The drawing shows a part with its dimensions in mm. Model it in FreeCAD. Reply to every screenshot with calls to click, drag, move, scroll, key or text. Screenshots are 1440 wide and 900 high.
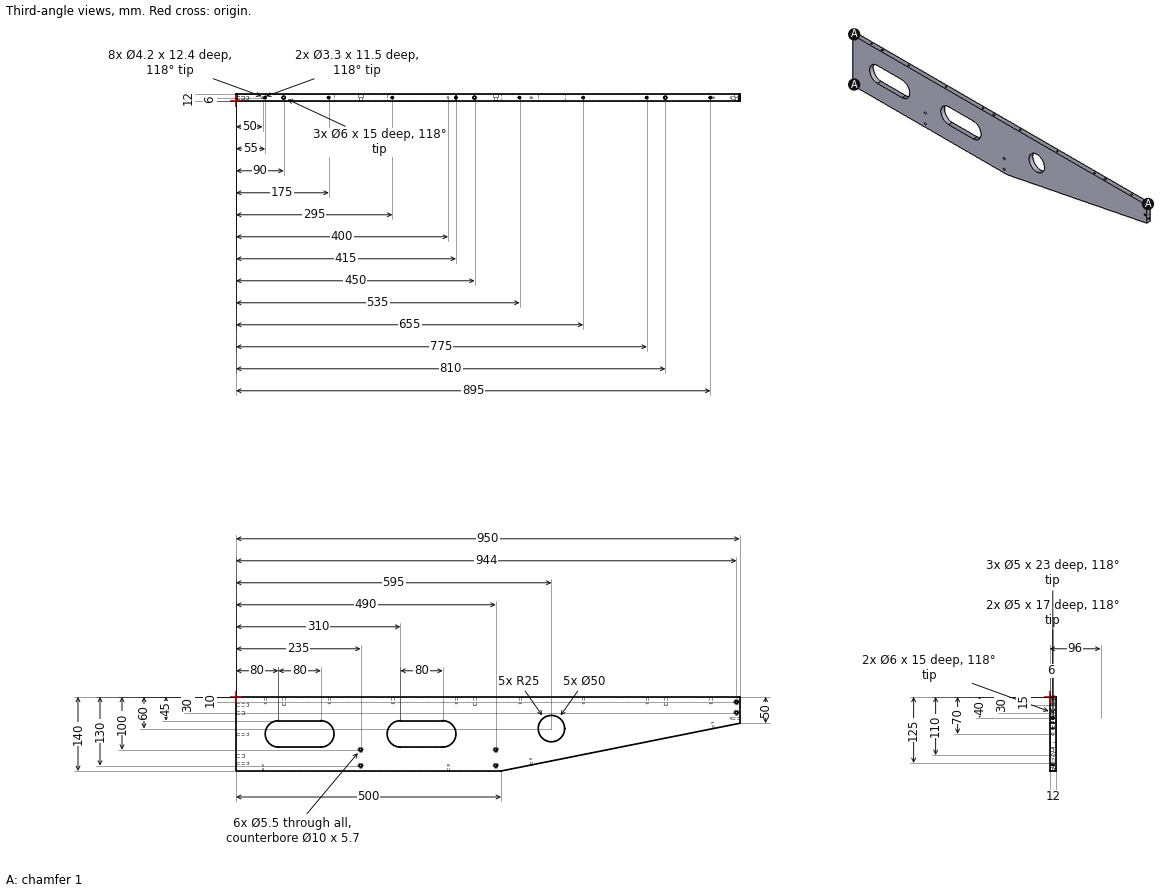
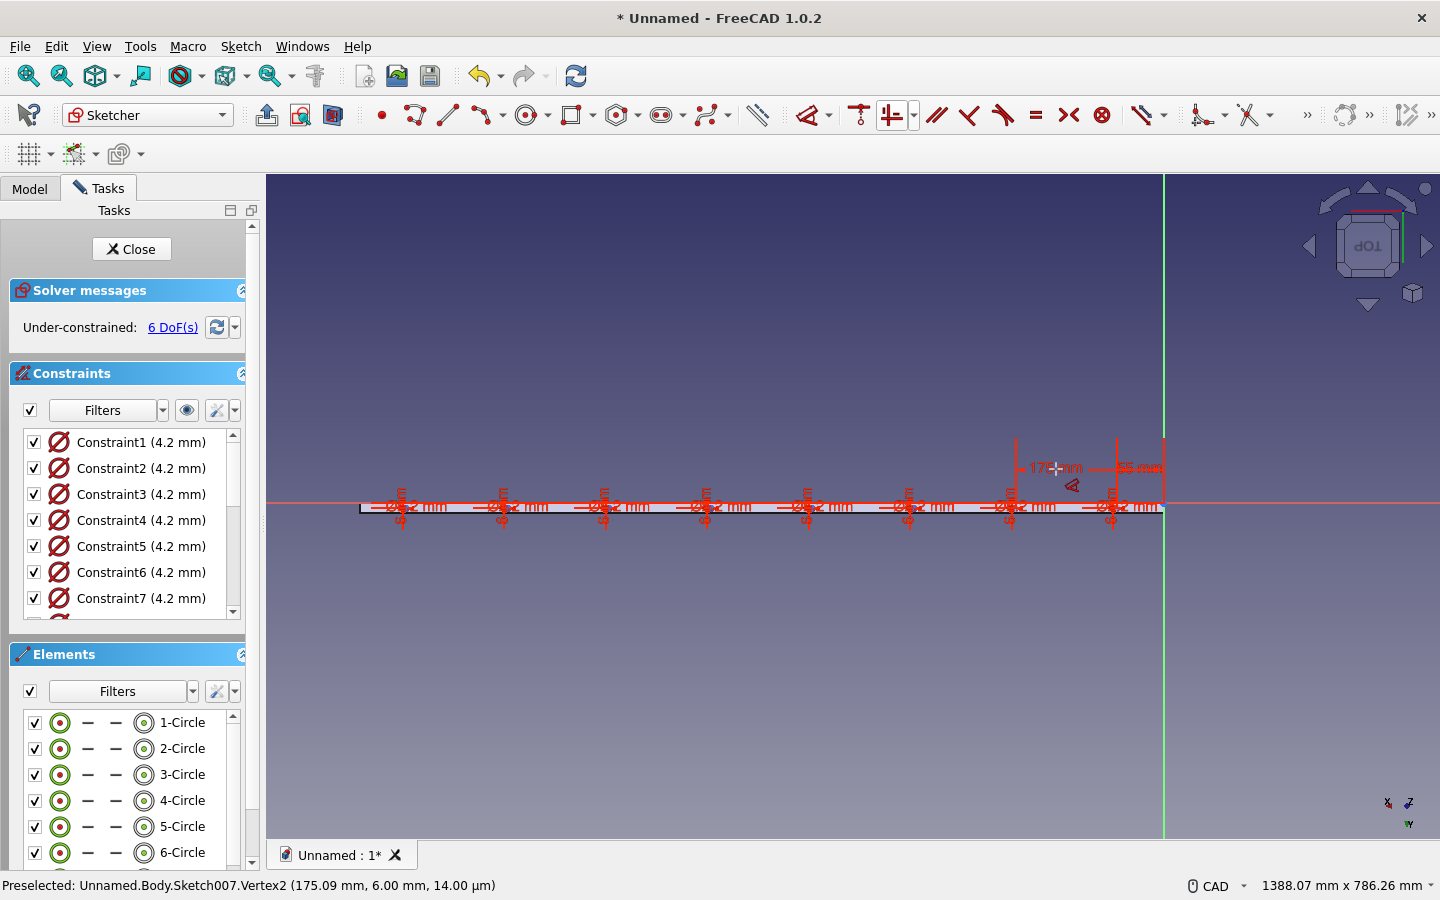
click(914, 508)
click(981, 469)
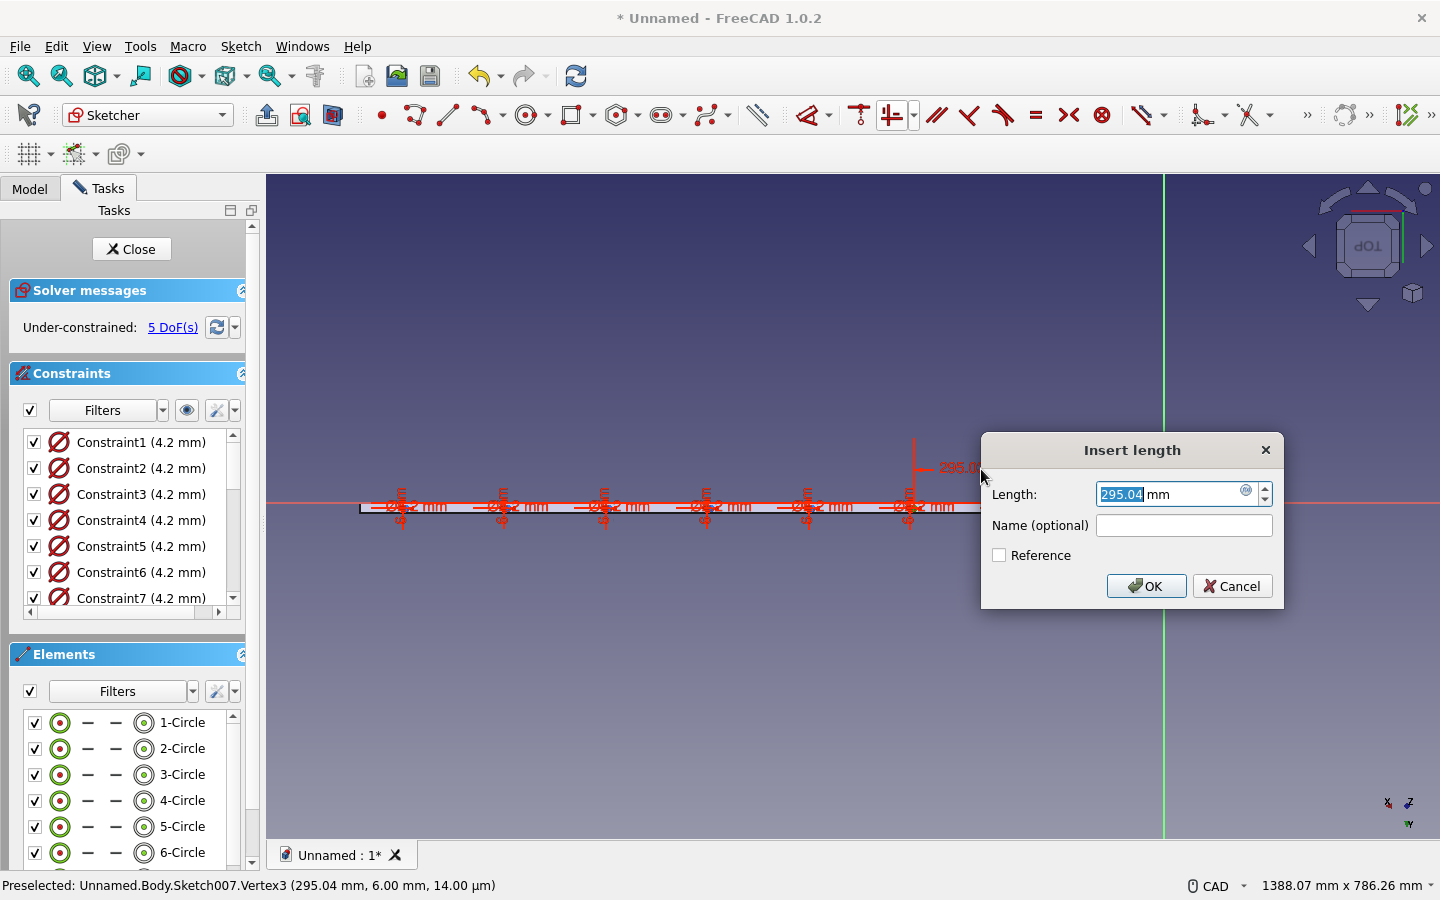
text(295)
key(Return)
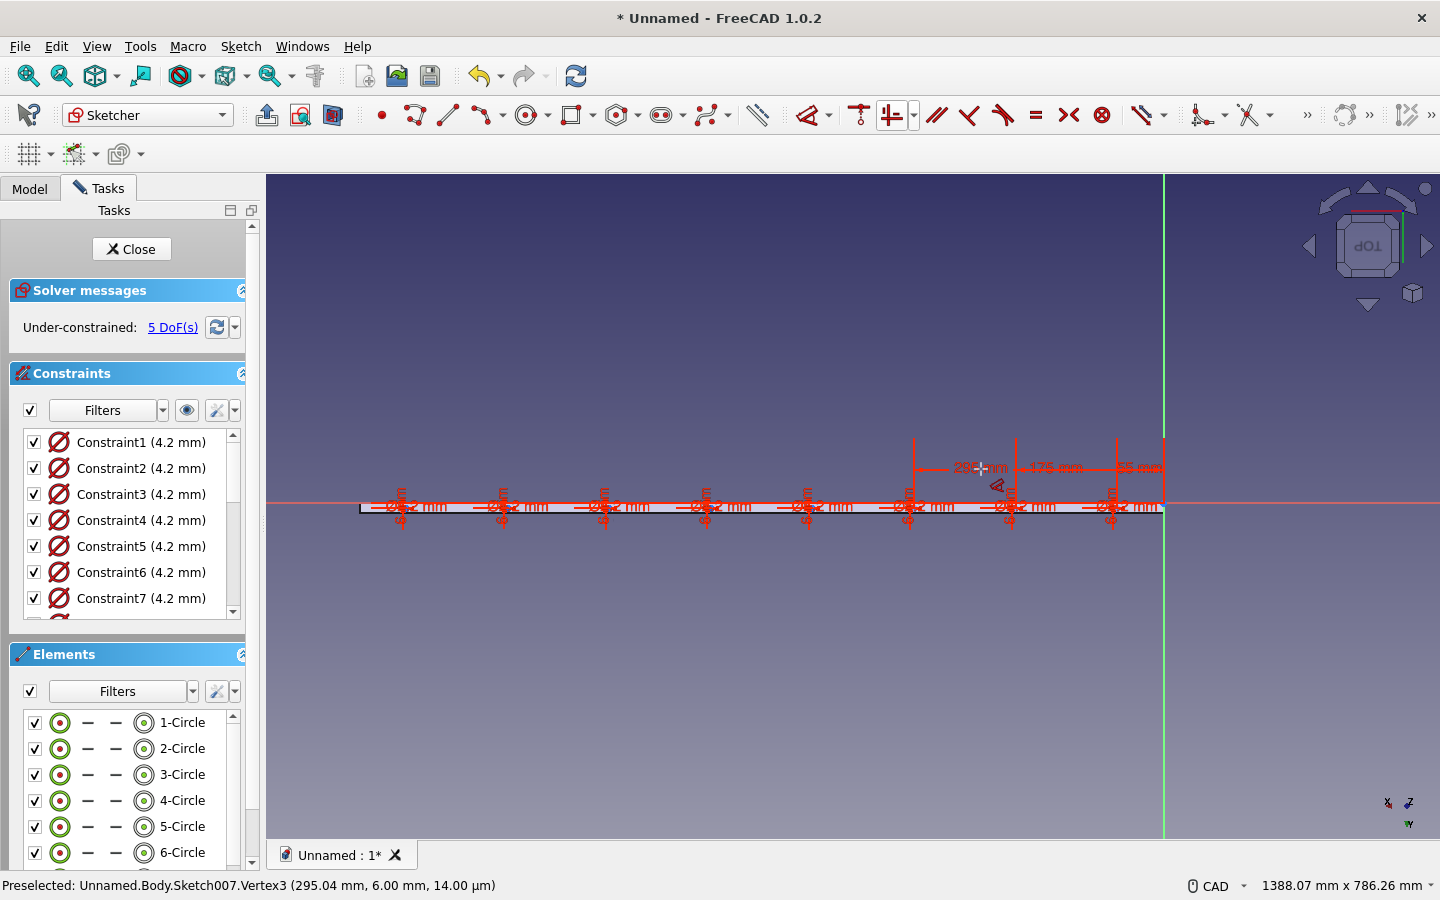
click(813, 508)
click(907, 469)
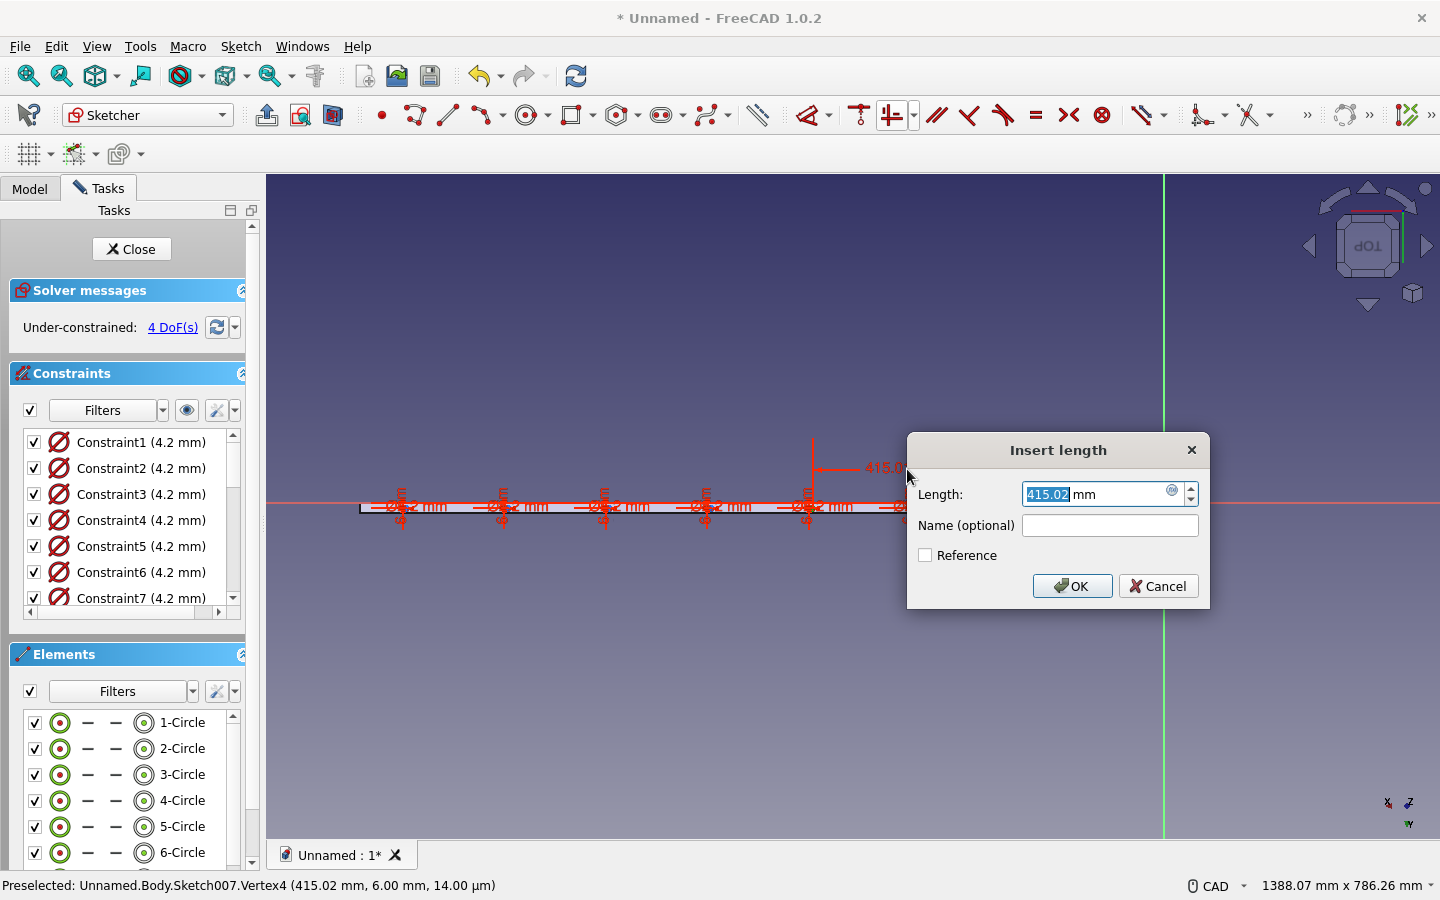
text(415)
key(Return)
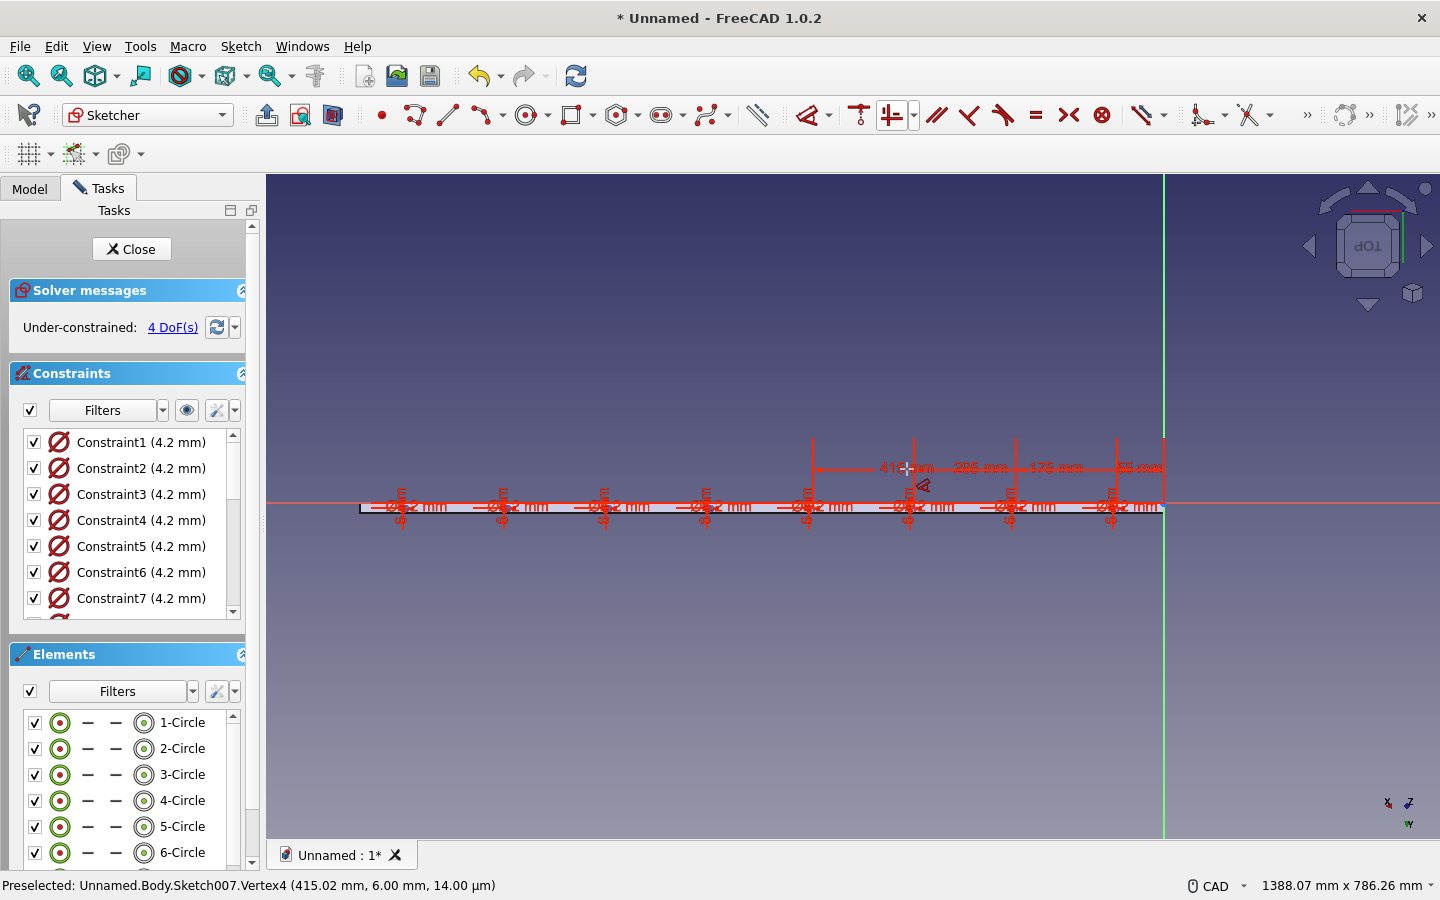
click(711, 508)
click(833, 469)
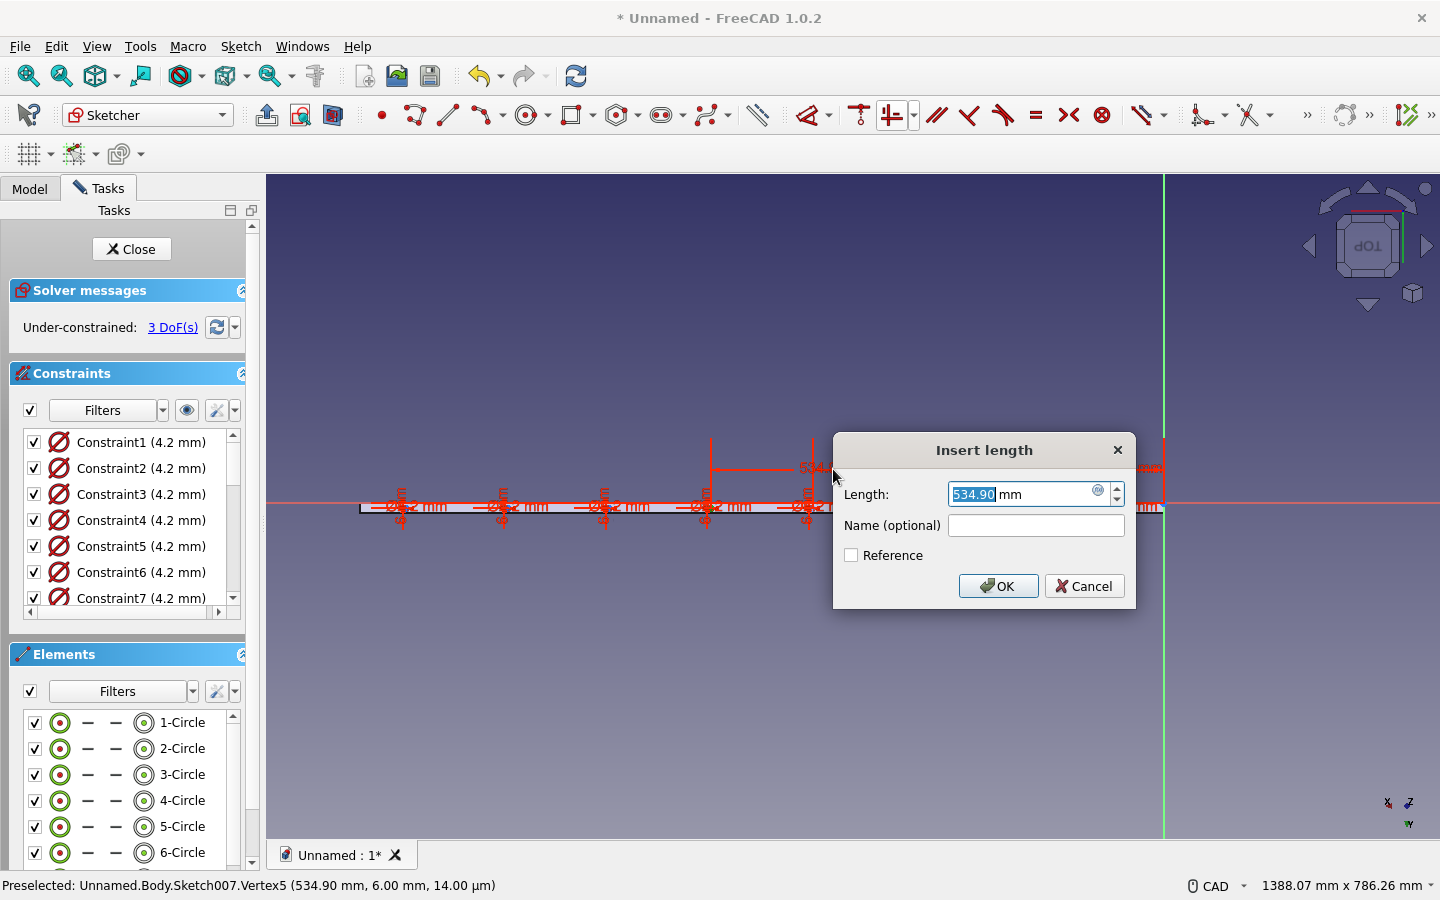
text(535)
key(Return)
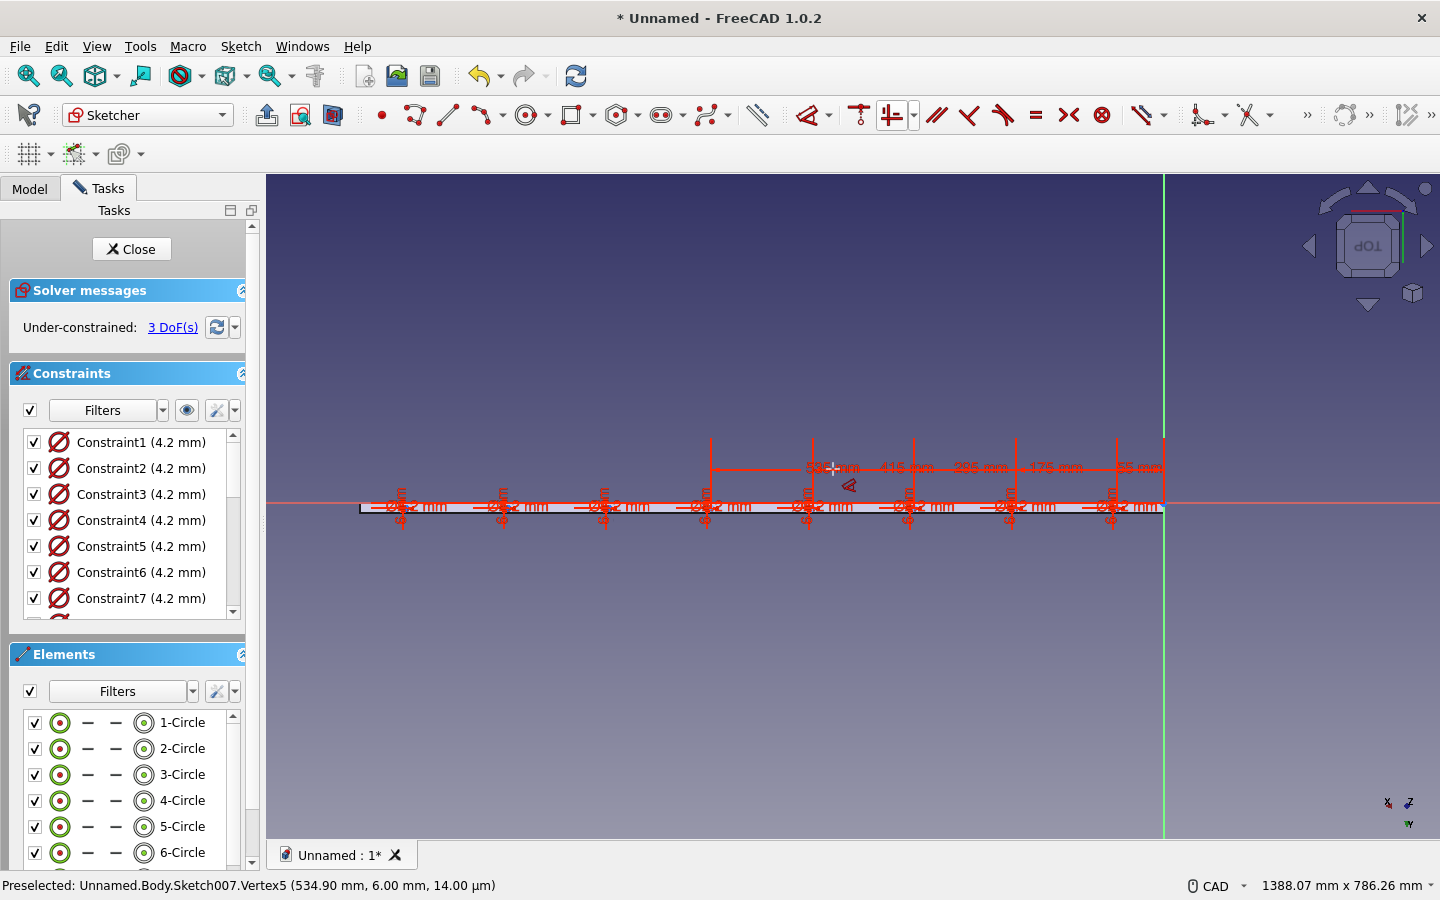
click(610, 508)
click(759, 469)